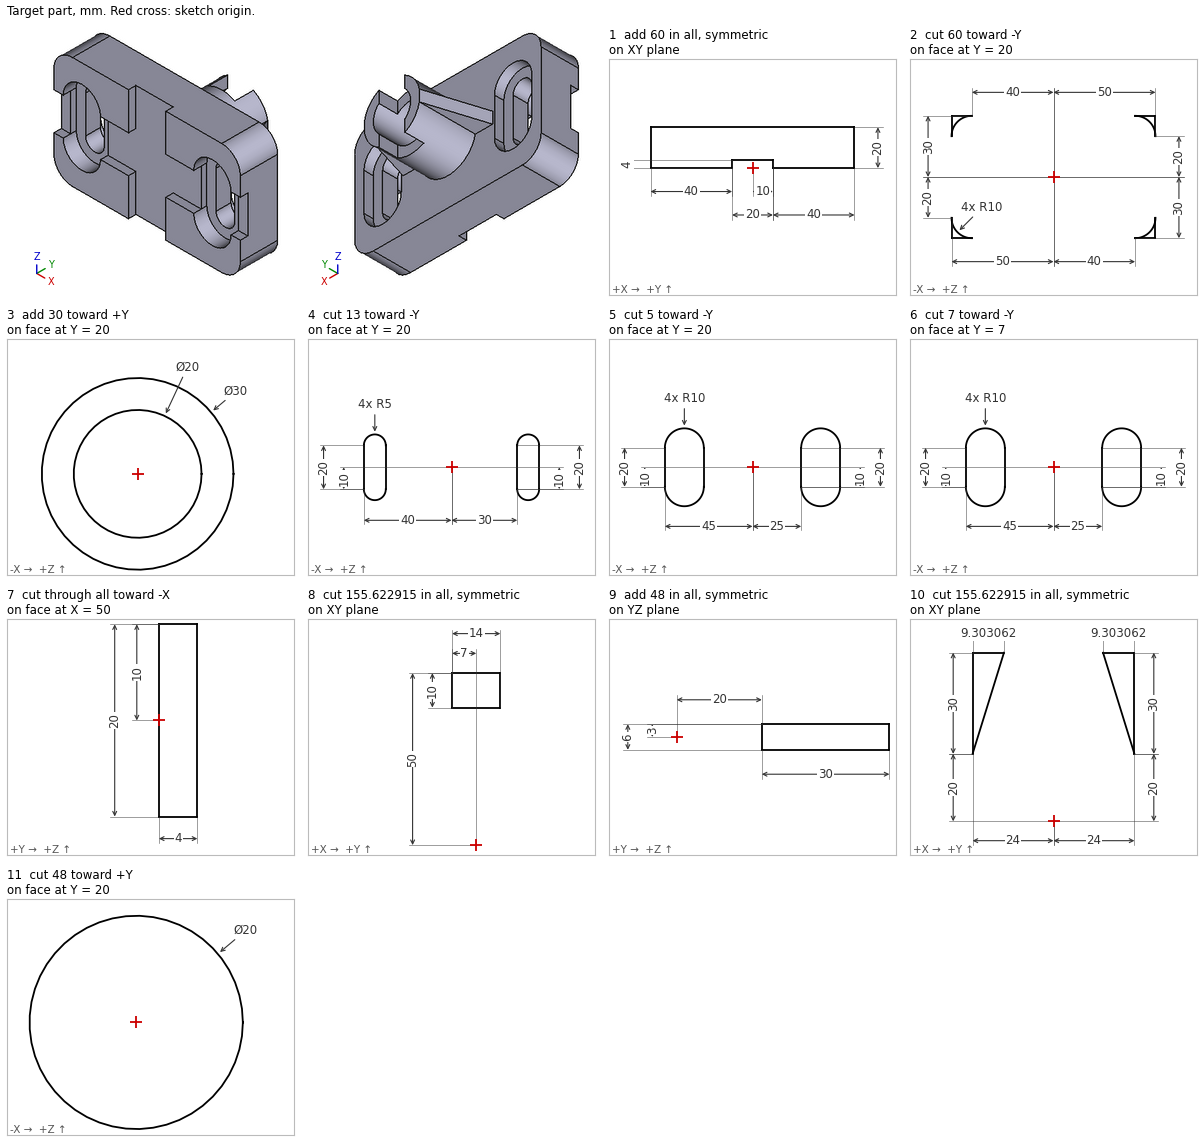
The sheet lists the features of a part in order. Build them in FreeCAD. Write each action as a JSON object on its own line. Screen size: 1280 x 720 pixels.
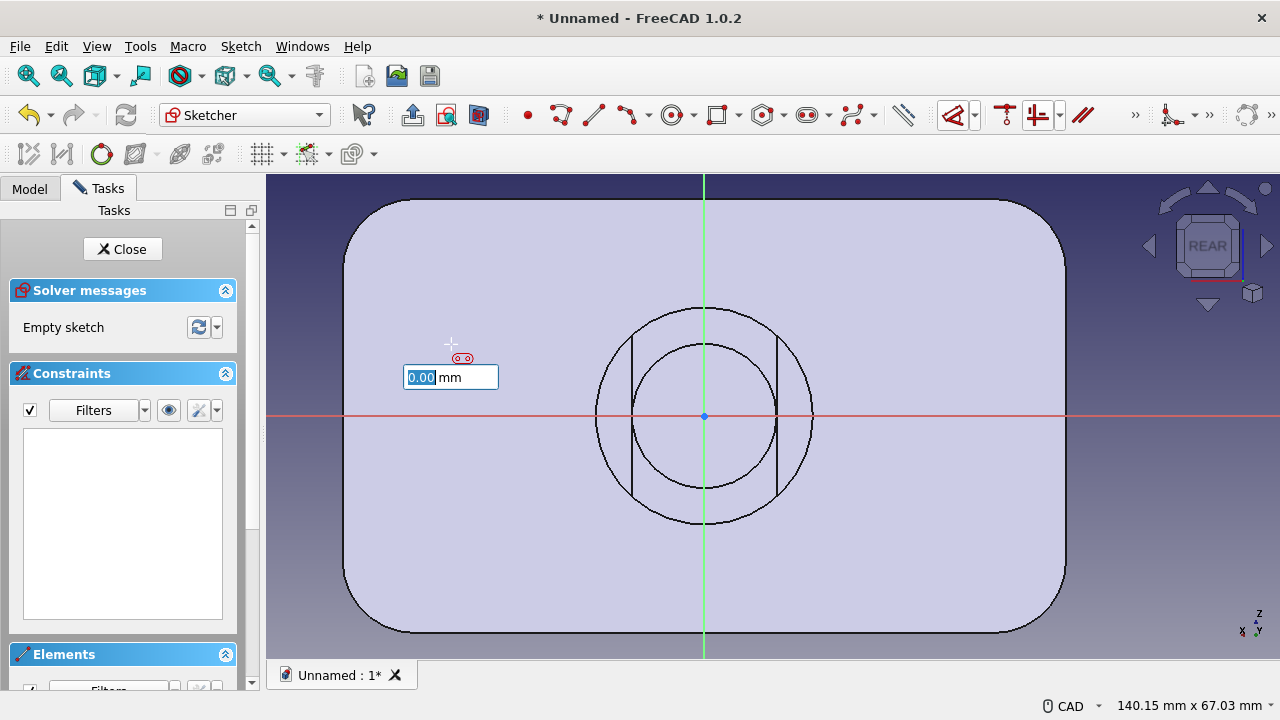
{"action": "left_click", "coordinate": [487, 438]}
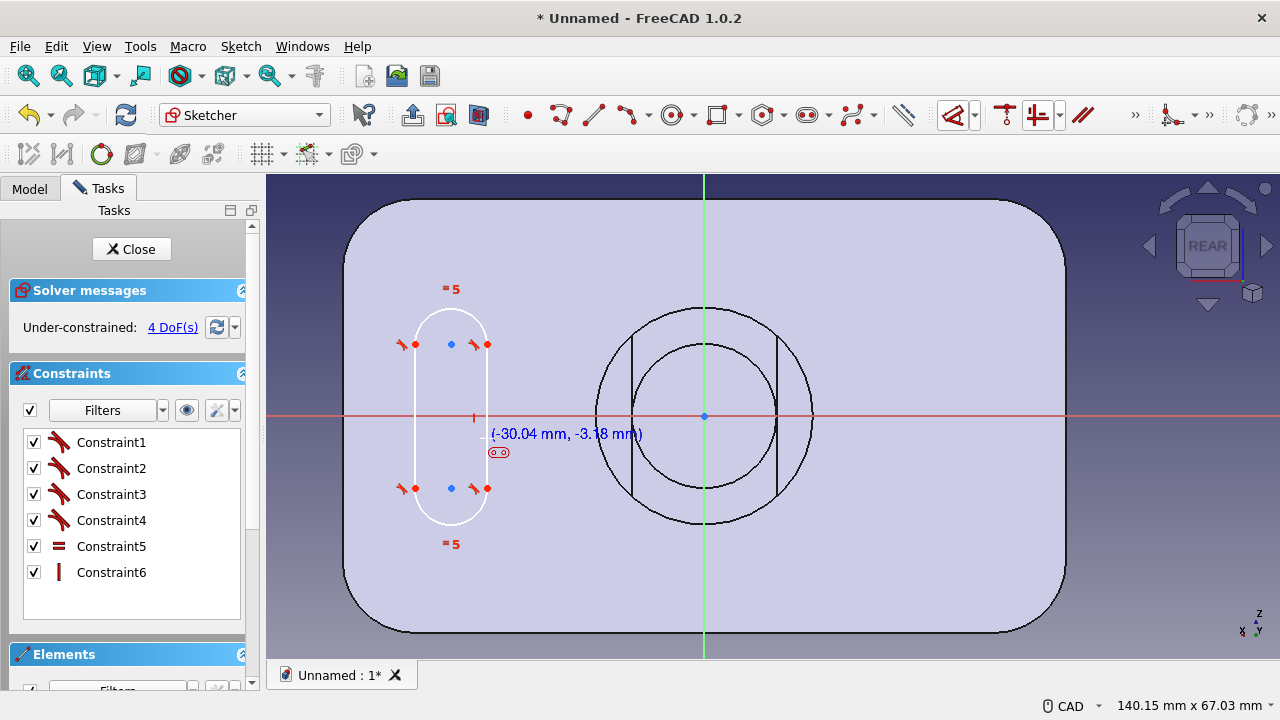
{"action": "left_click", "coordinate": [958, 488]}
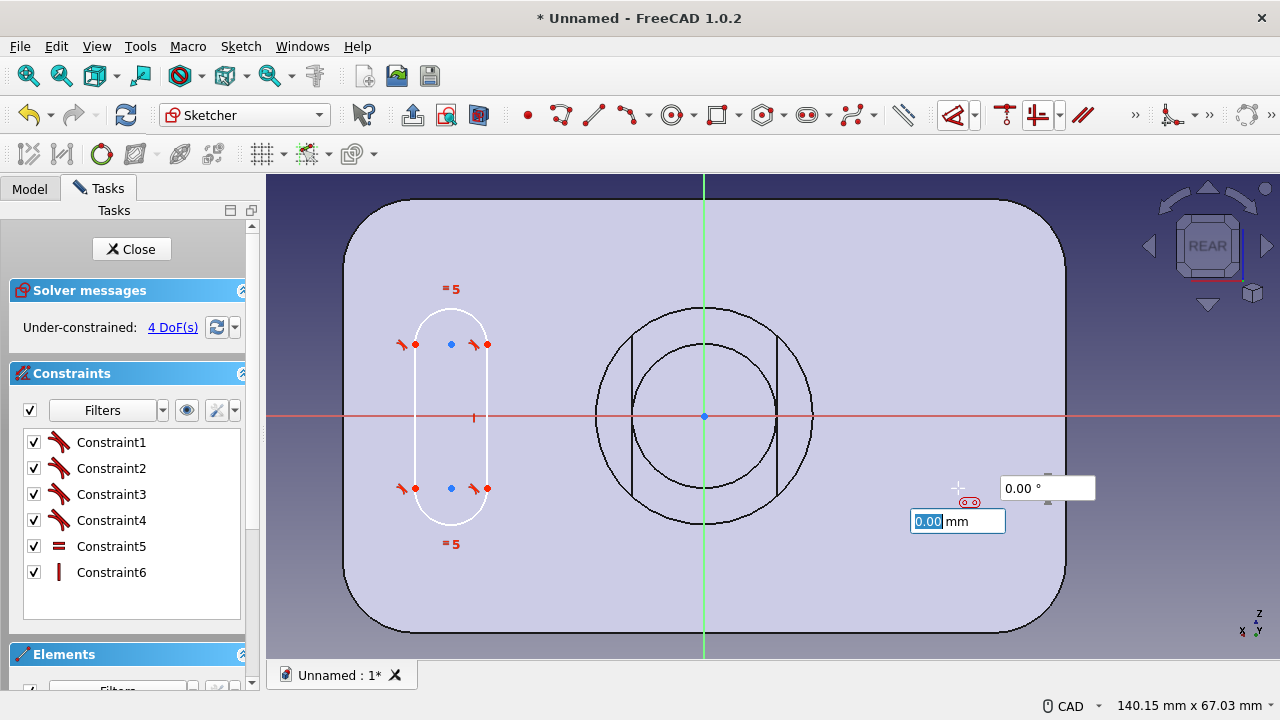
{"action": "left_click", "coordinate": [958, 344]}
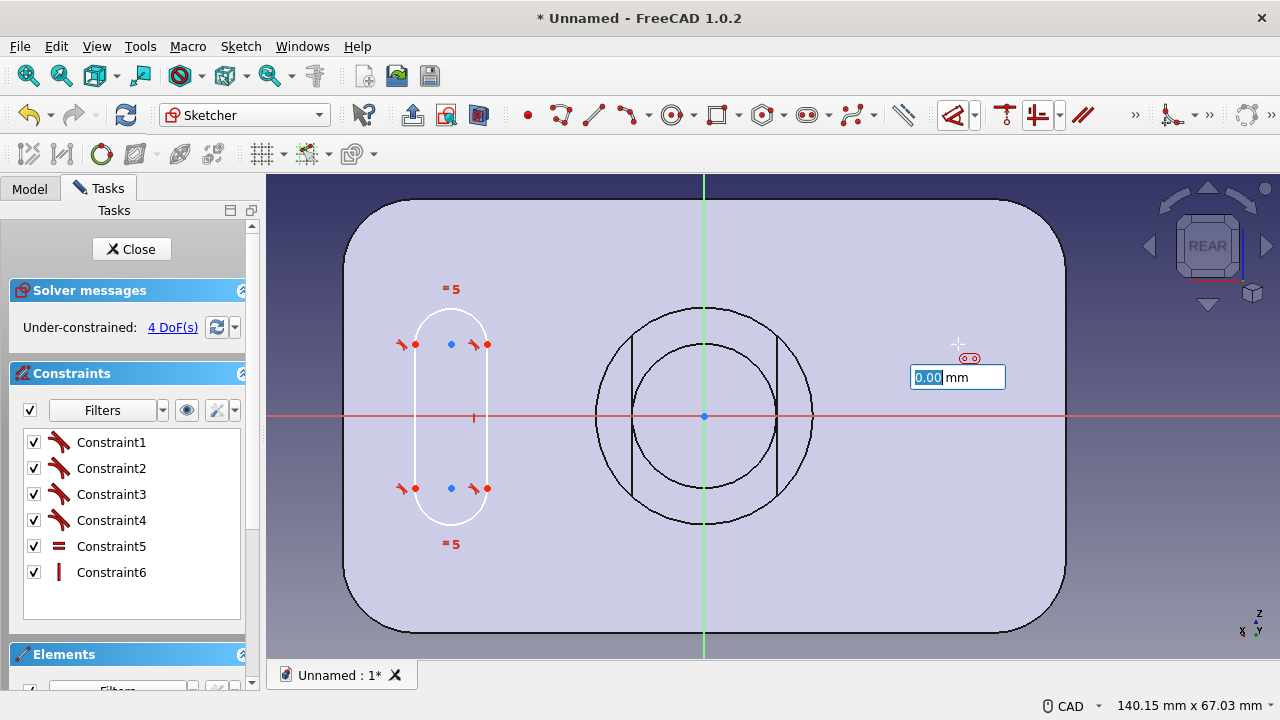
{"action": "left_click", "coordinate": [921, 394]}
{"action": "key", "text": "Escape"}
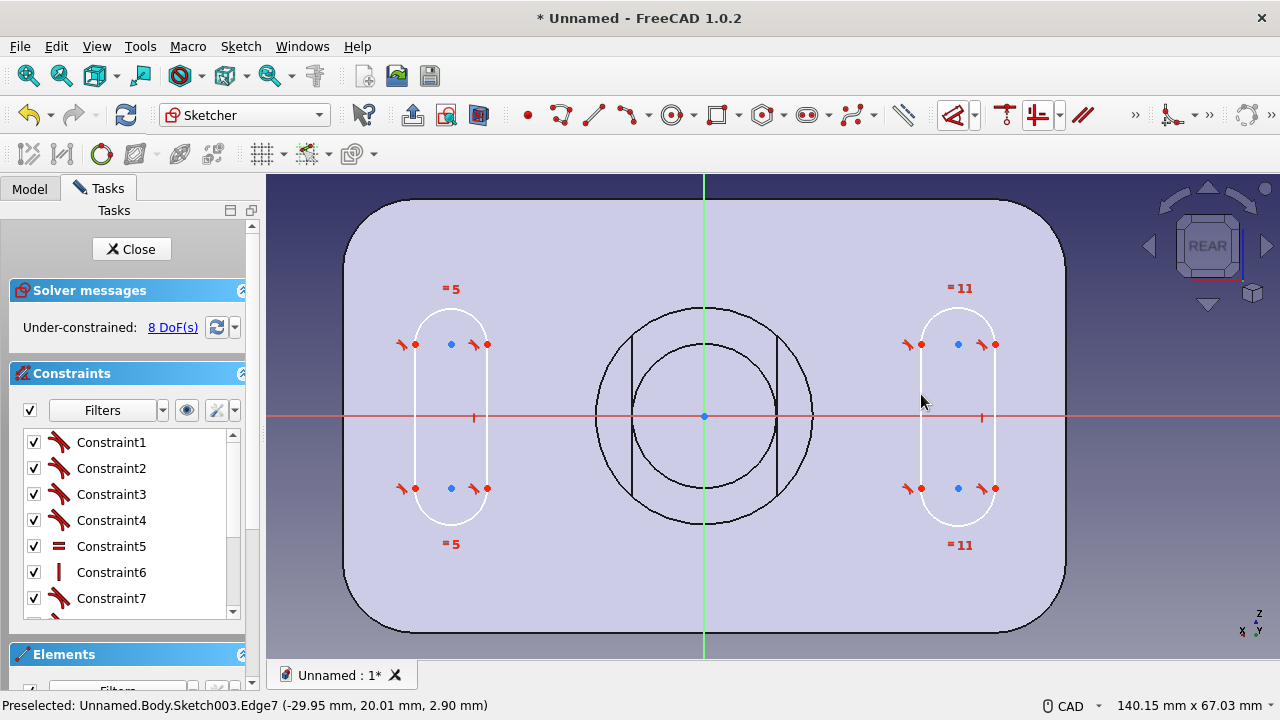
{"action": "left_click", "coordinate": [430, 518]}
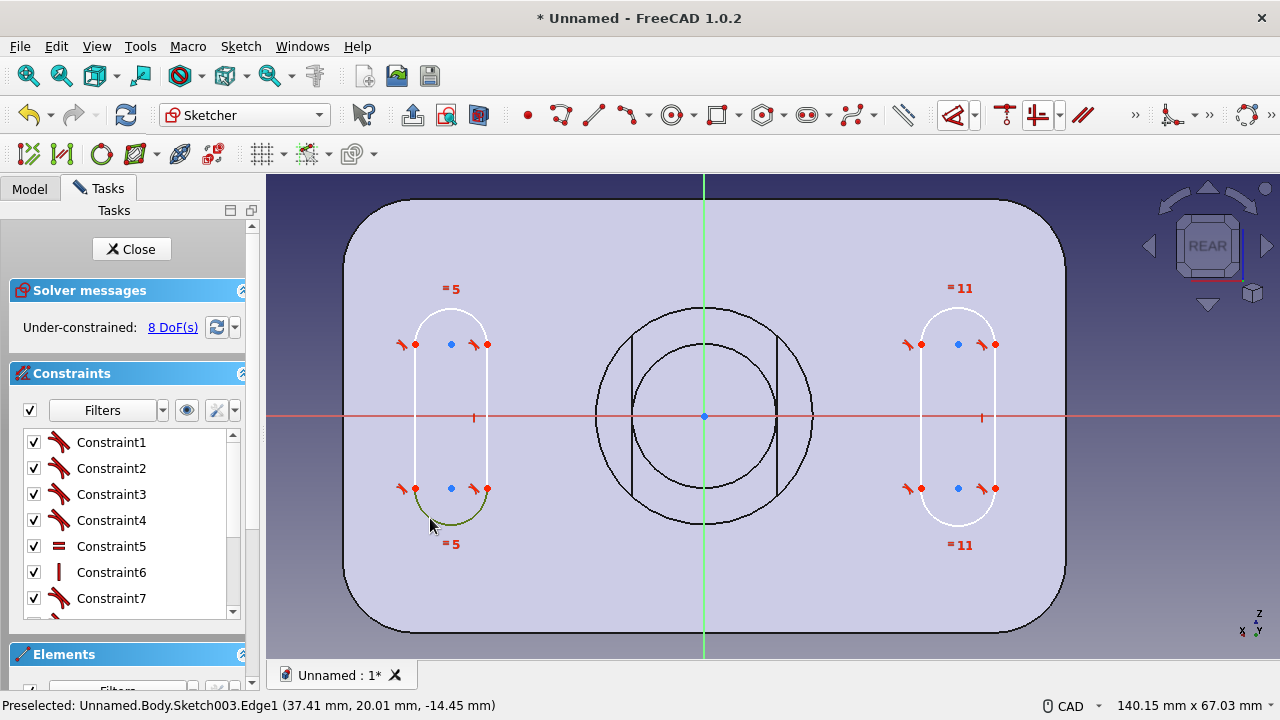
{"action": "left_click", "coordinate": [936, 519]}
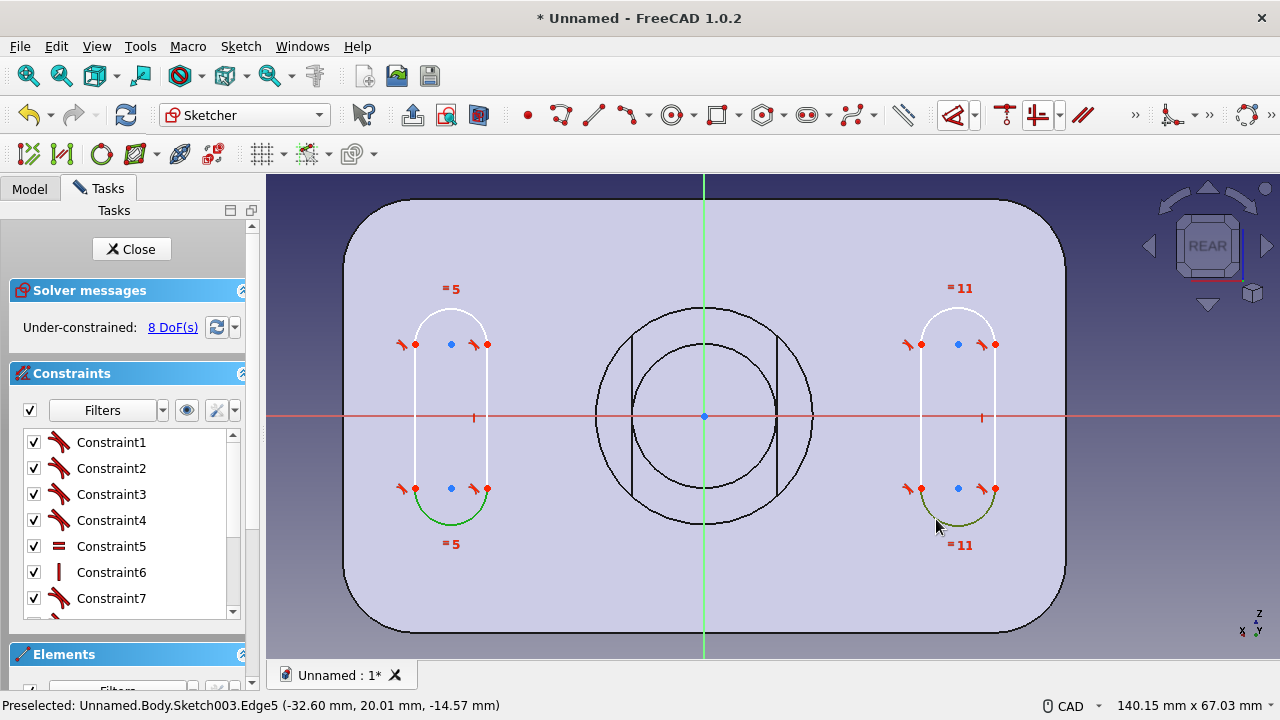
{"action": "key", "text": "e"}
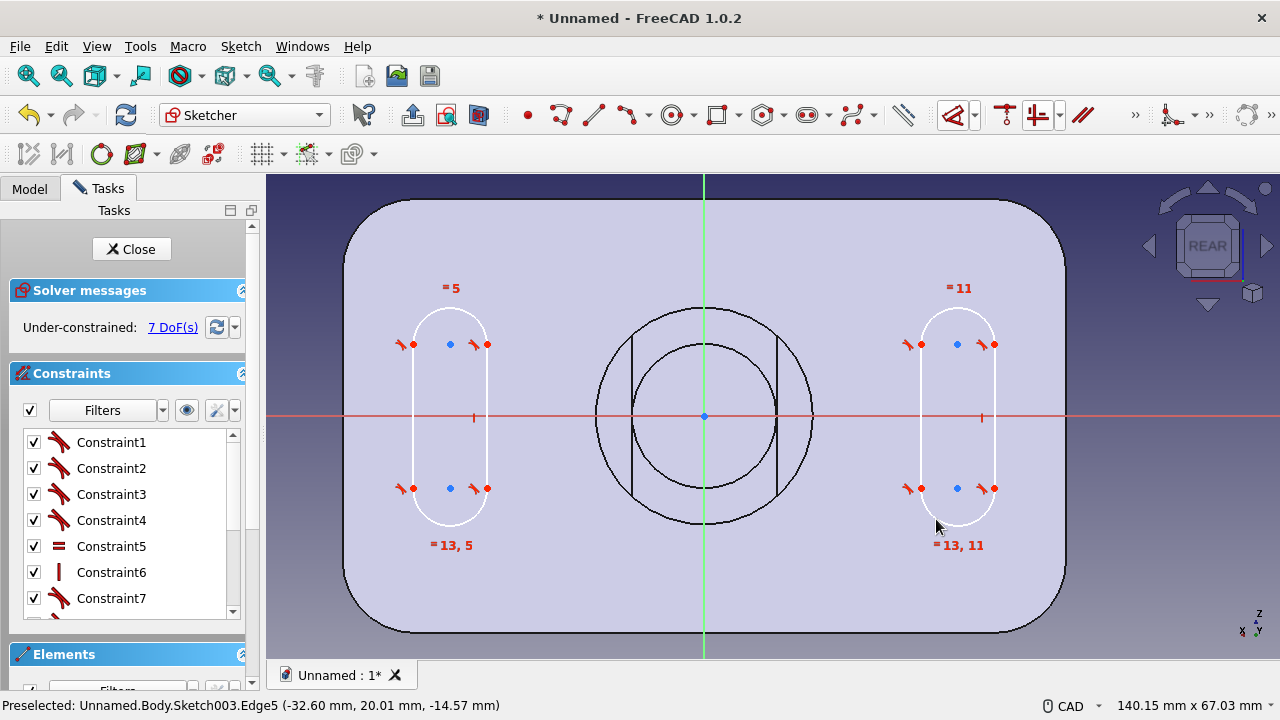
{"action": "left_click", "coordinate": [429, 519]}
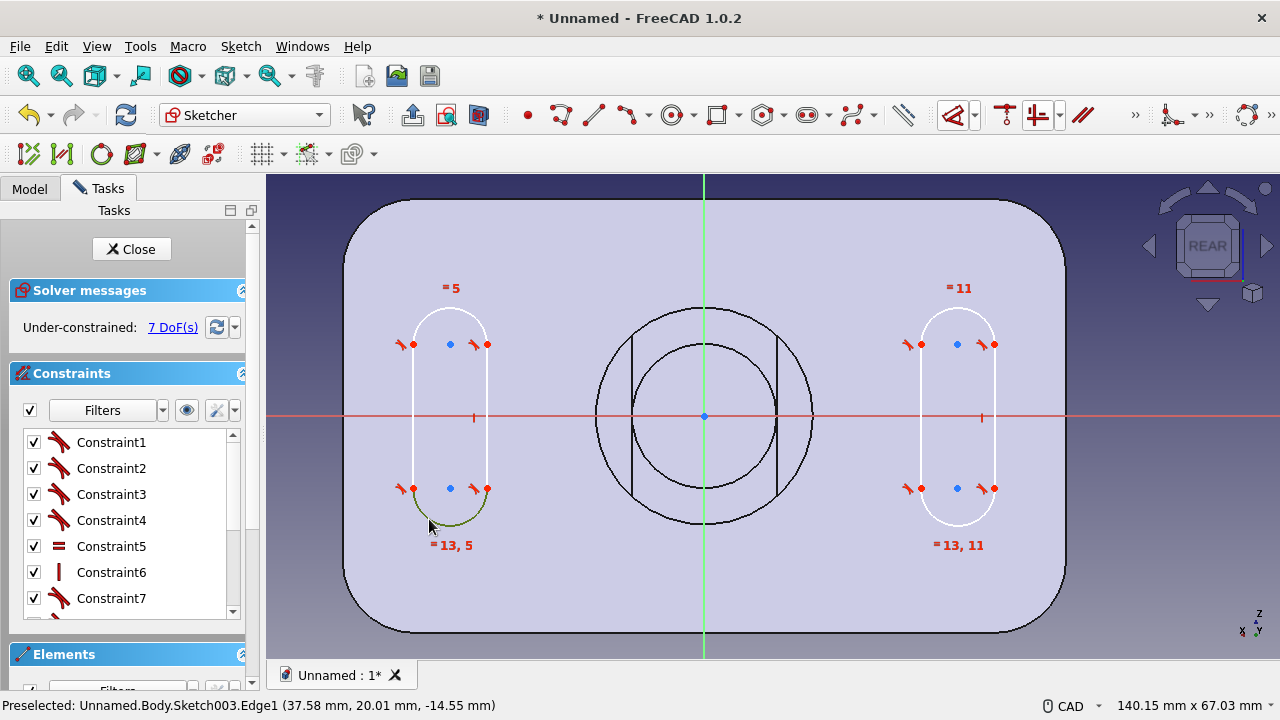
{"action": "key", "text": "k r"}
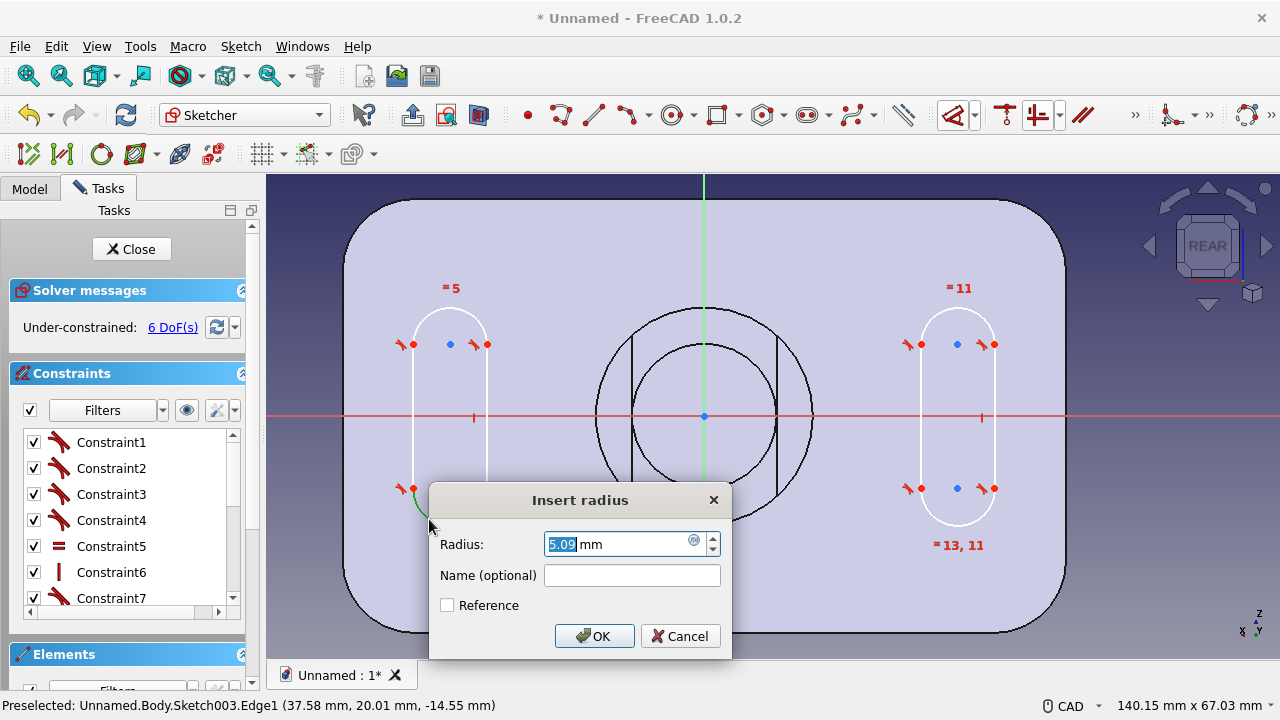
{"action": "type", "text": "5"}
{"action": "key", "text": "Return"}